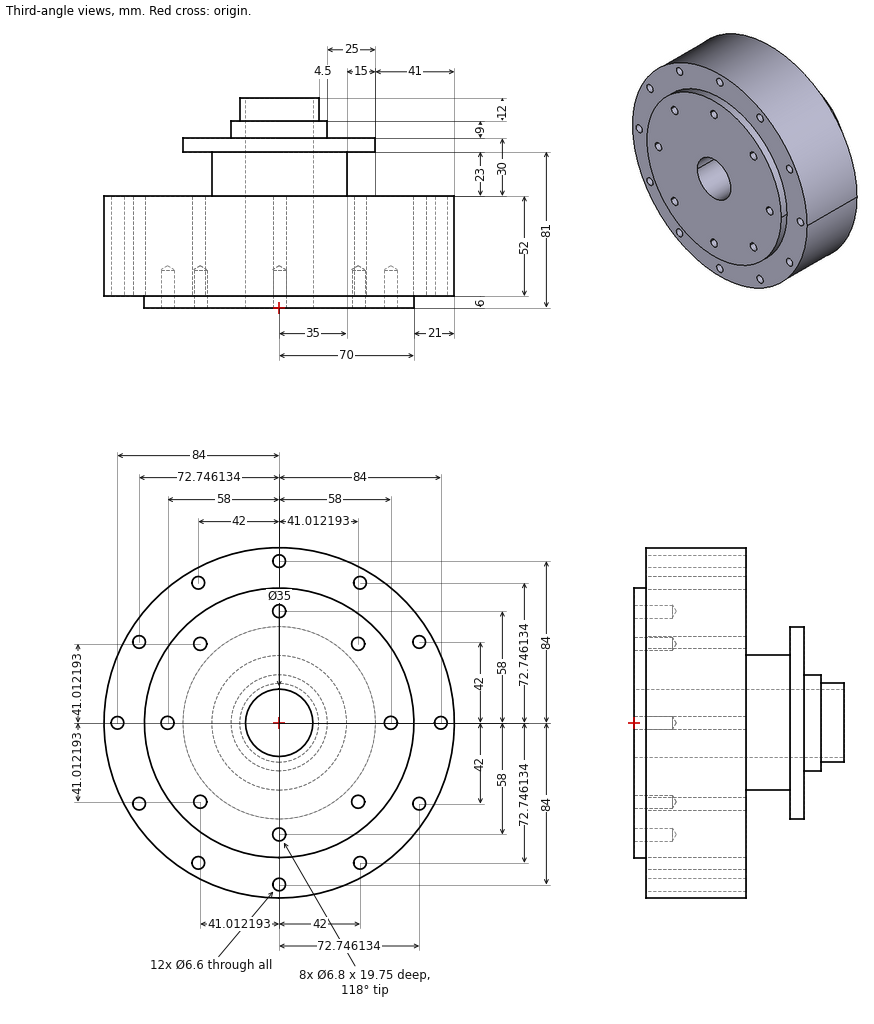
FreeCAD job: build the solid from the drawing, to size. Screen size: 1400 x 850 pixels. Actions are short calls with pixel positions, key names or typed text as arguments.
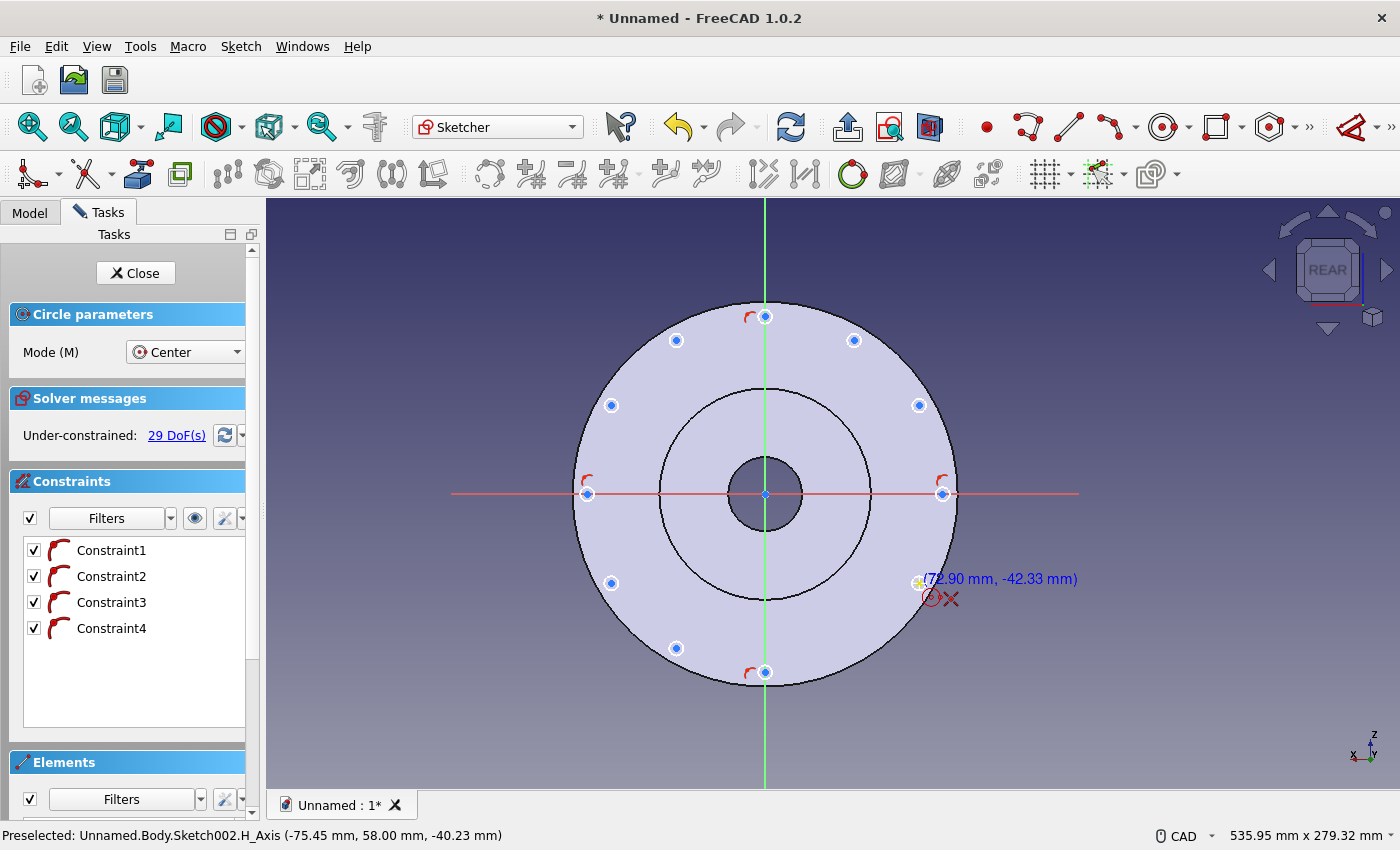
scroll(854, 648, up, 6)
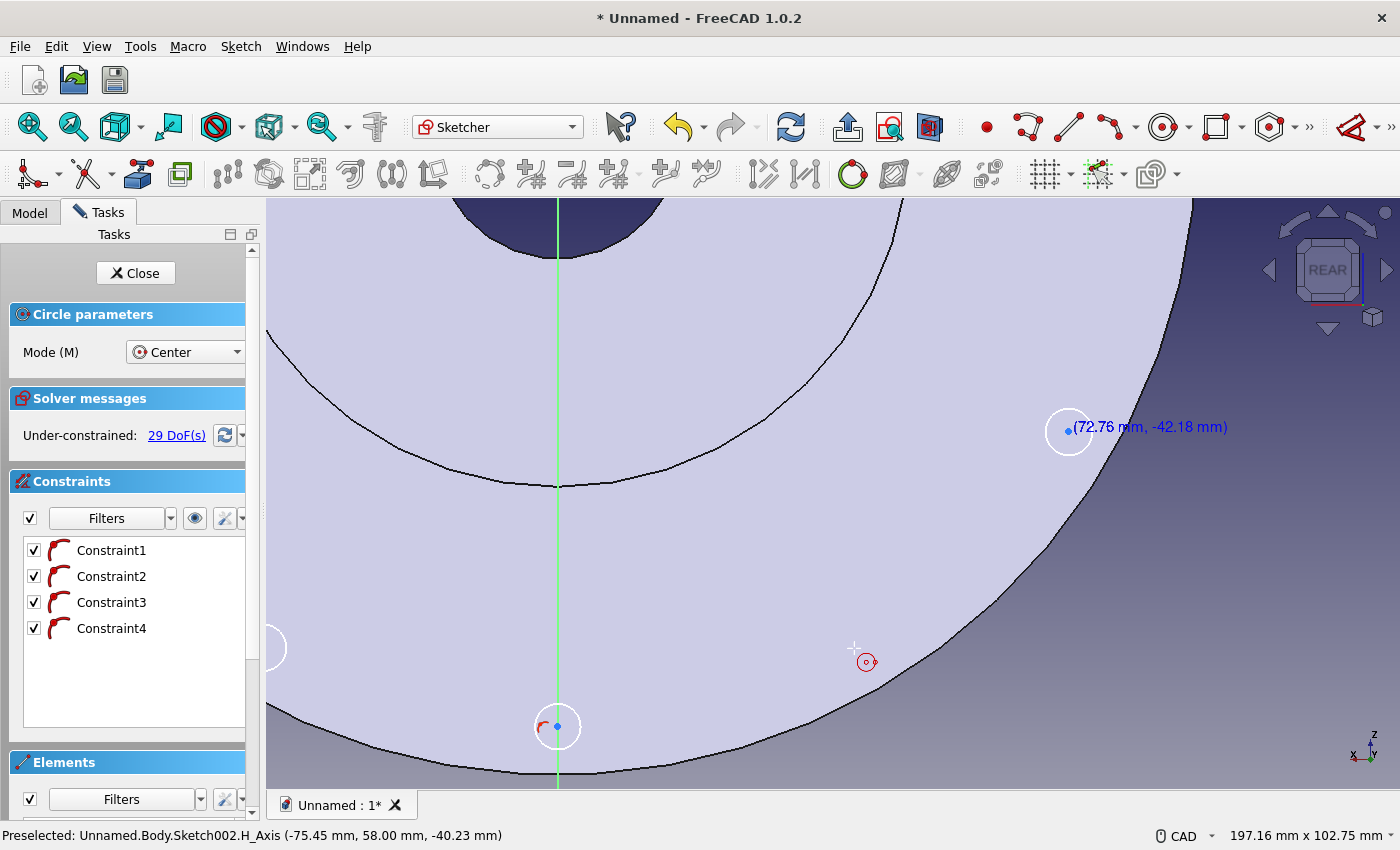
click(853, 647)
click(869, 630)
key(Escape)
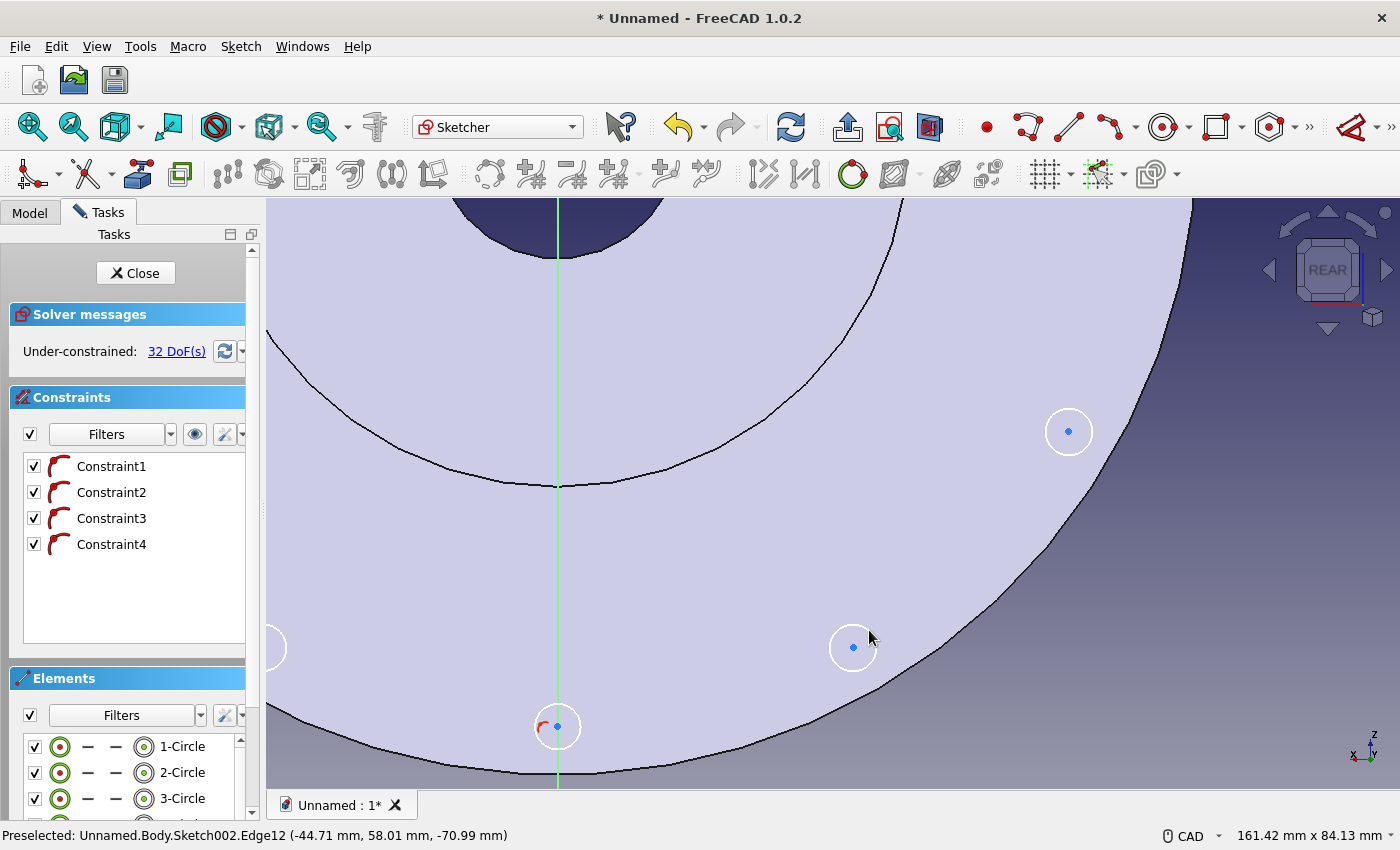
click(574, 711)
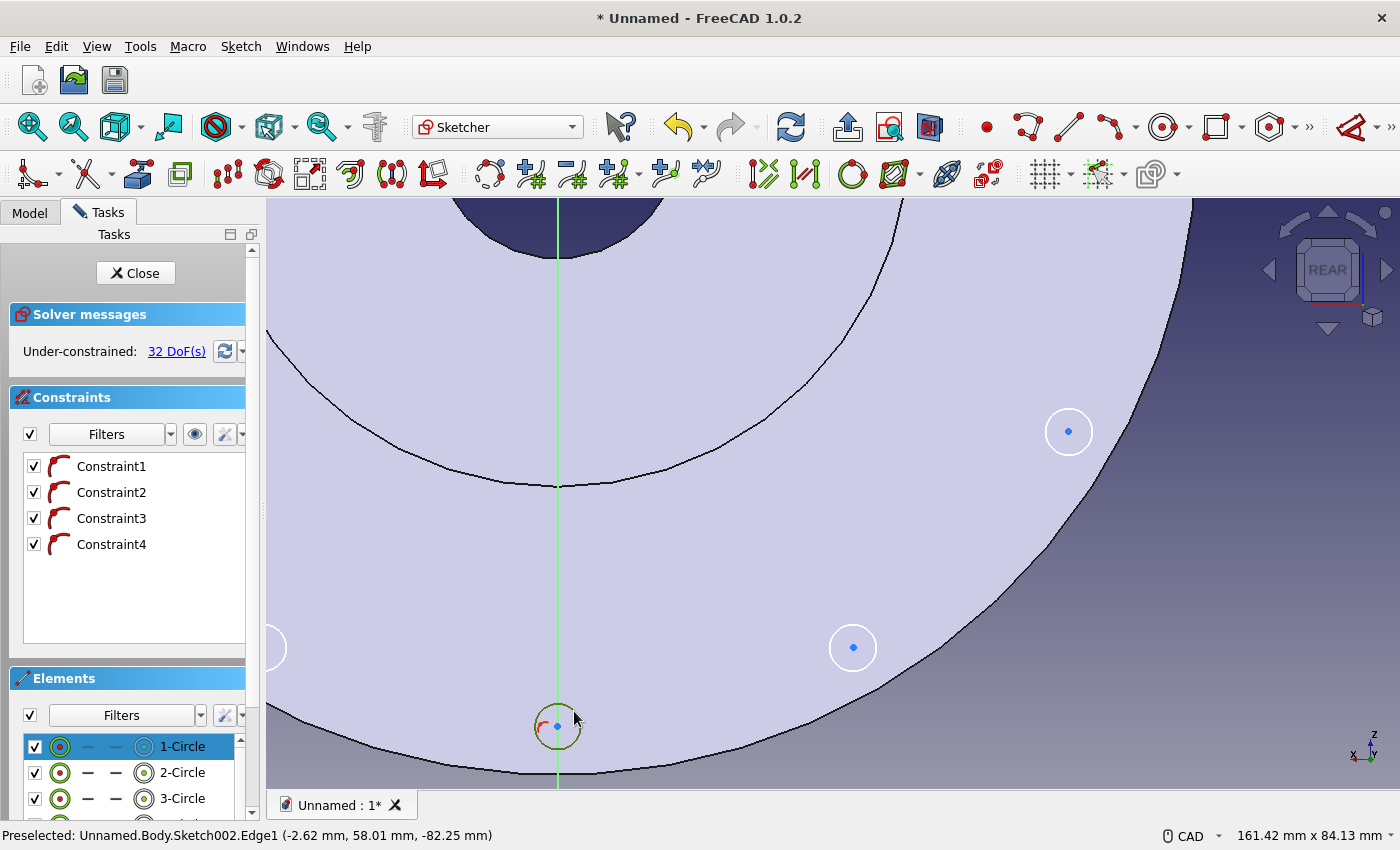
scroll(854, 648, down, 6)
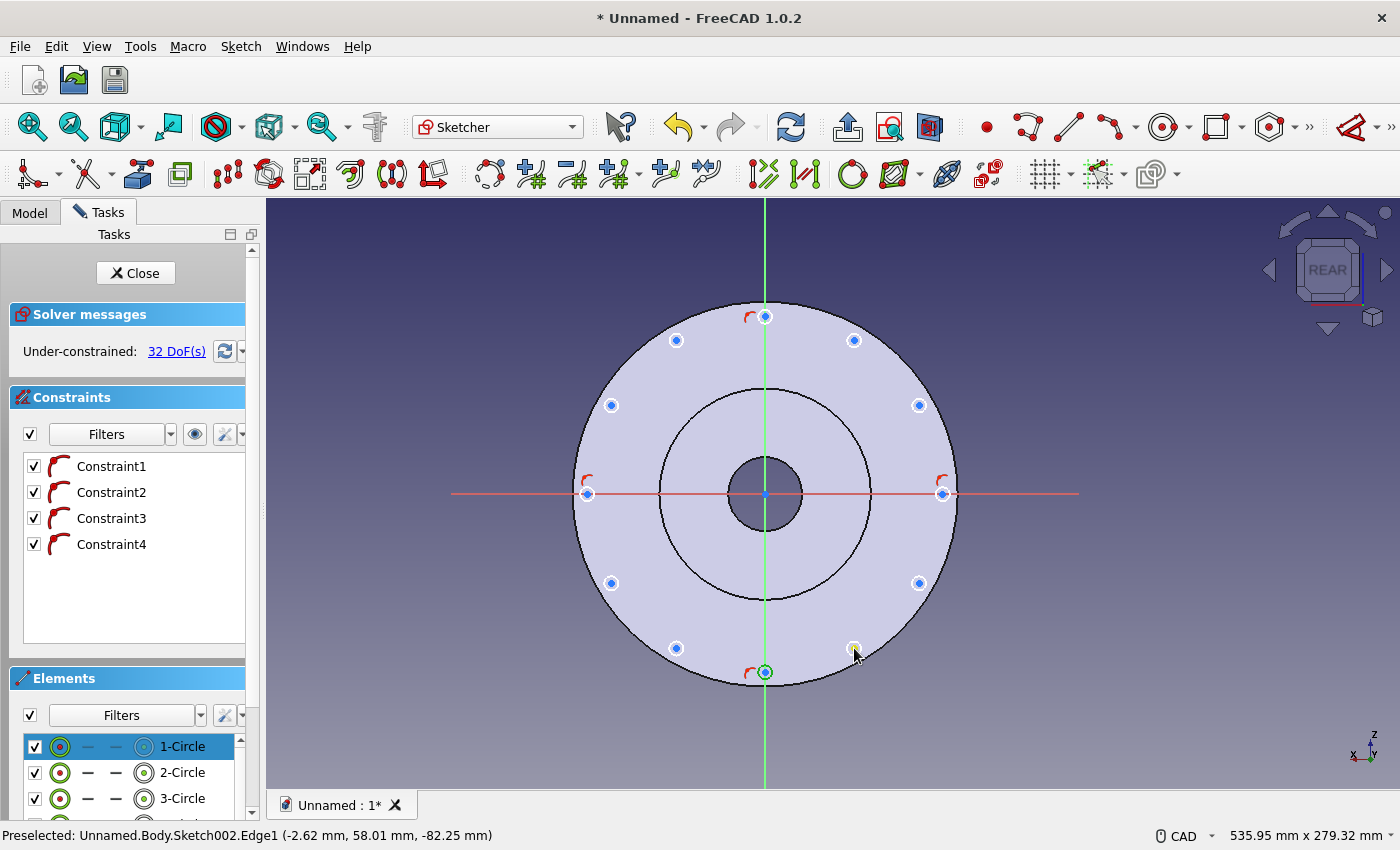
scroll(681, 643, up, 4)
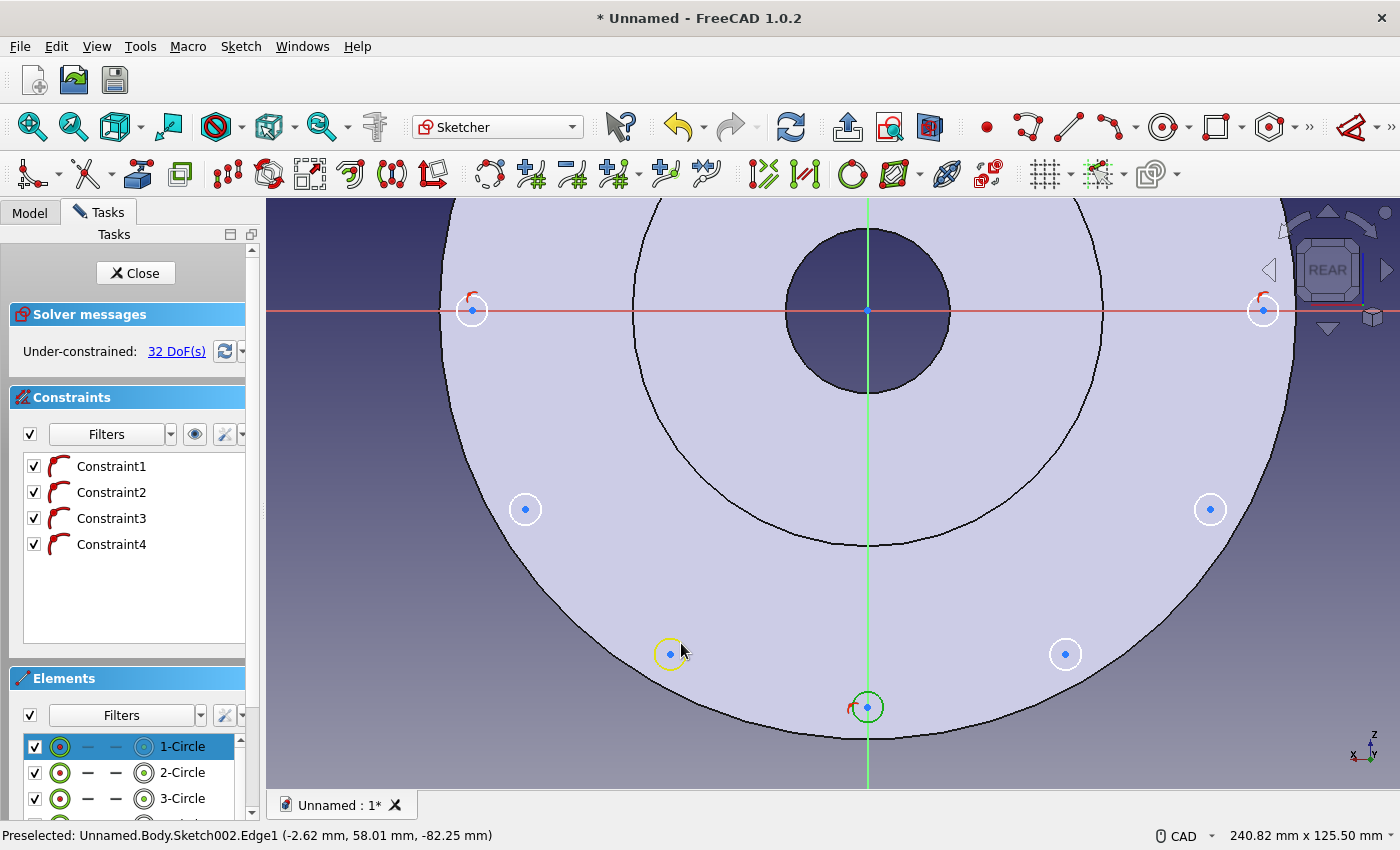
click(681, 643)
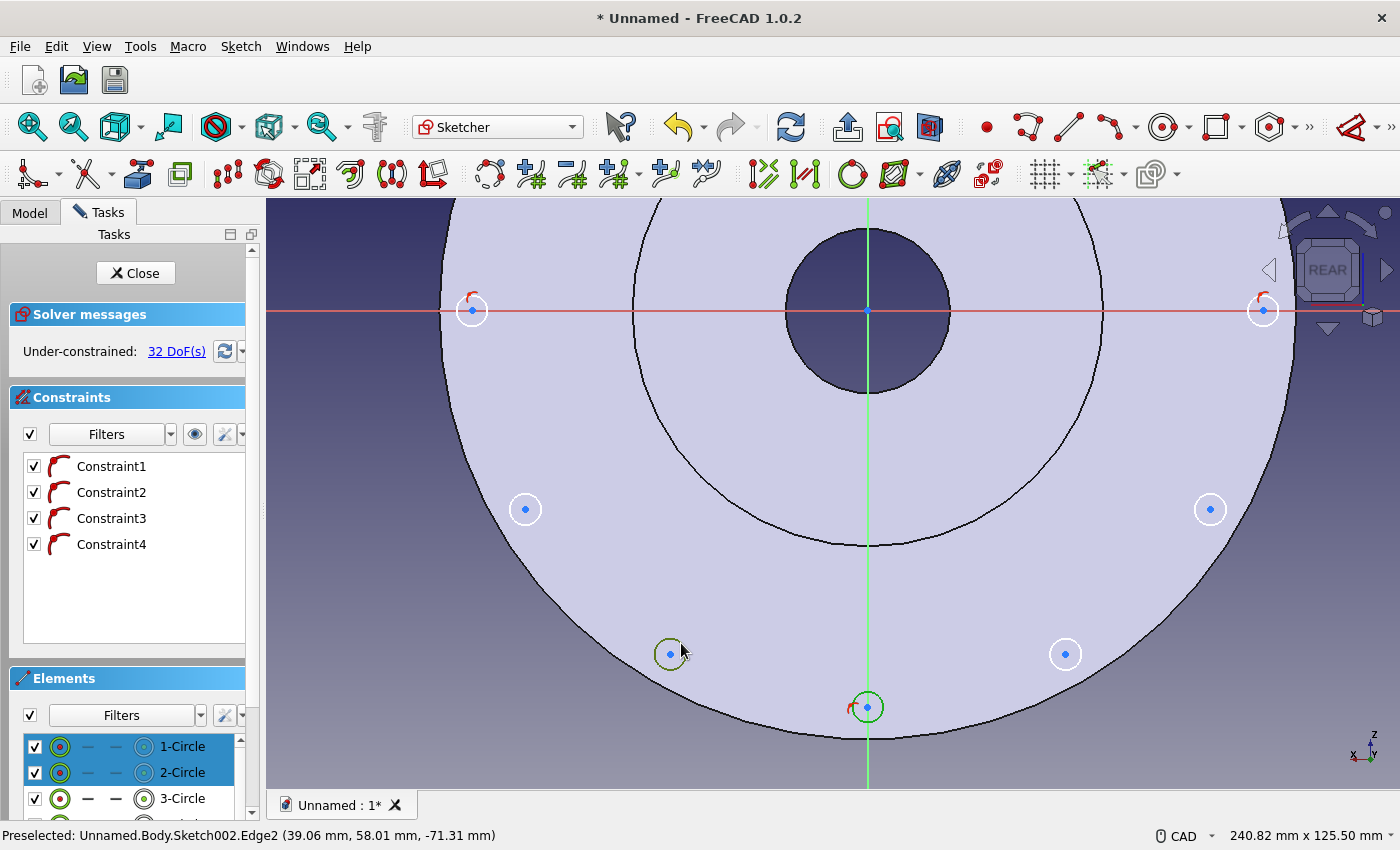
click(536, 498)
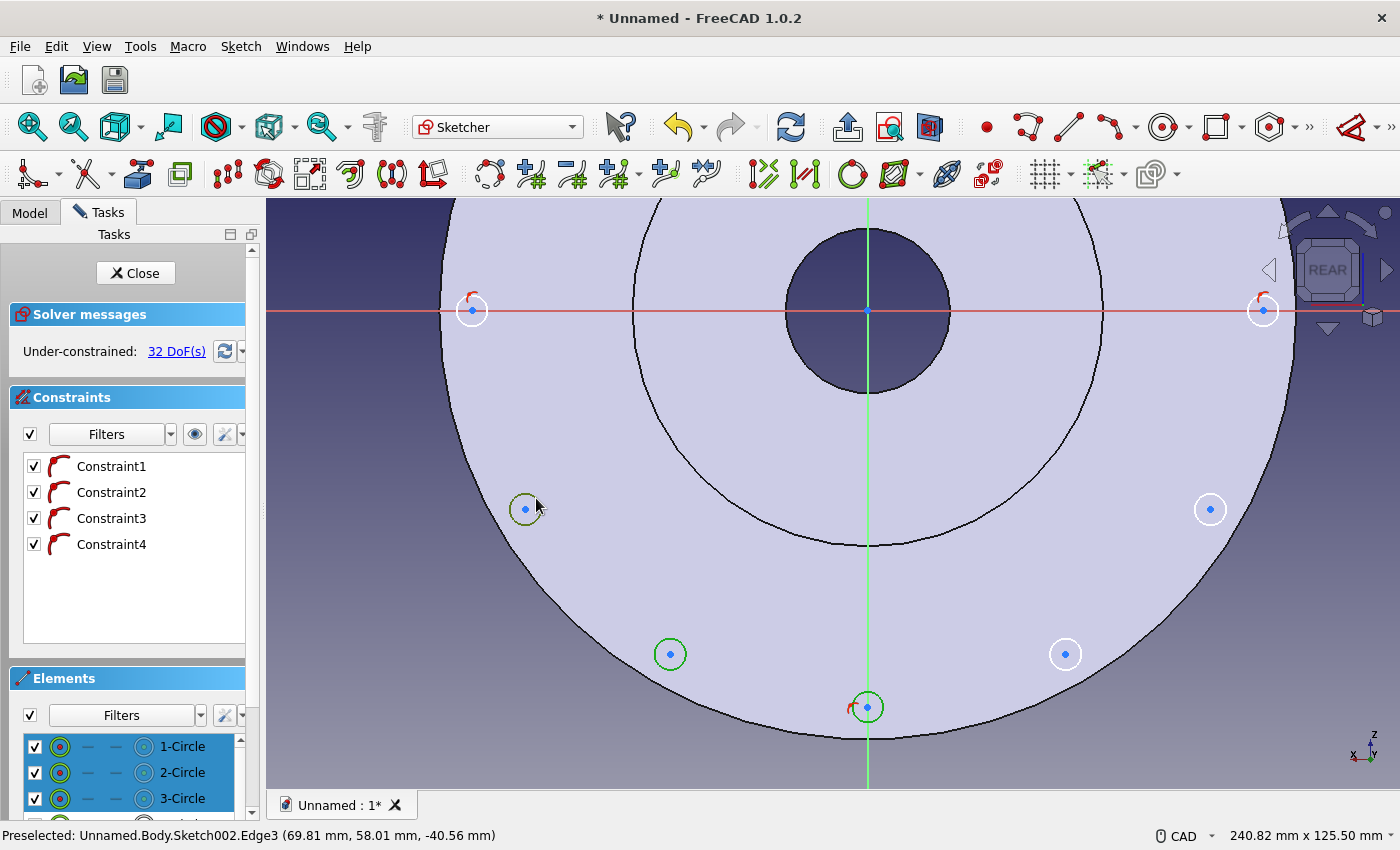
scroll(483, 300, up, 2)